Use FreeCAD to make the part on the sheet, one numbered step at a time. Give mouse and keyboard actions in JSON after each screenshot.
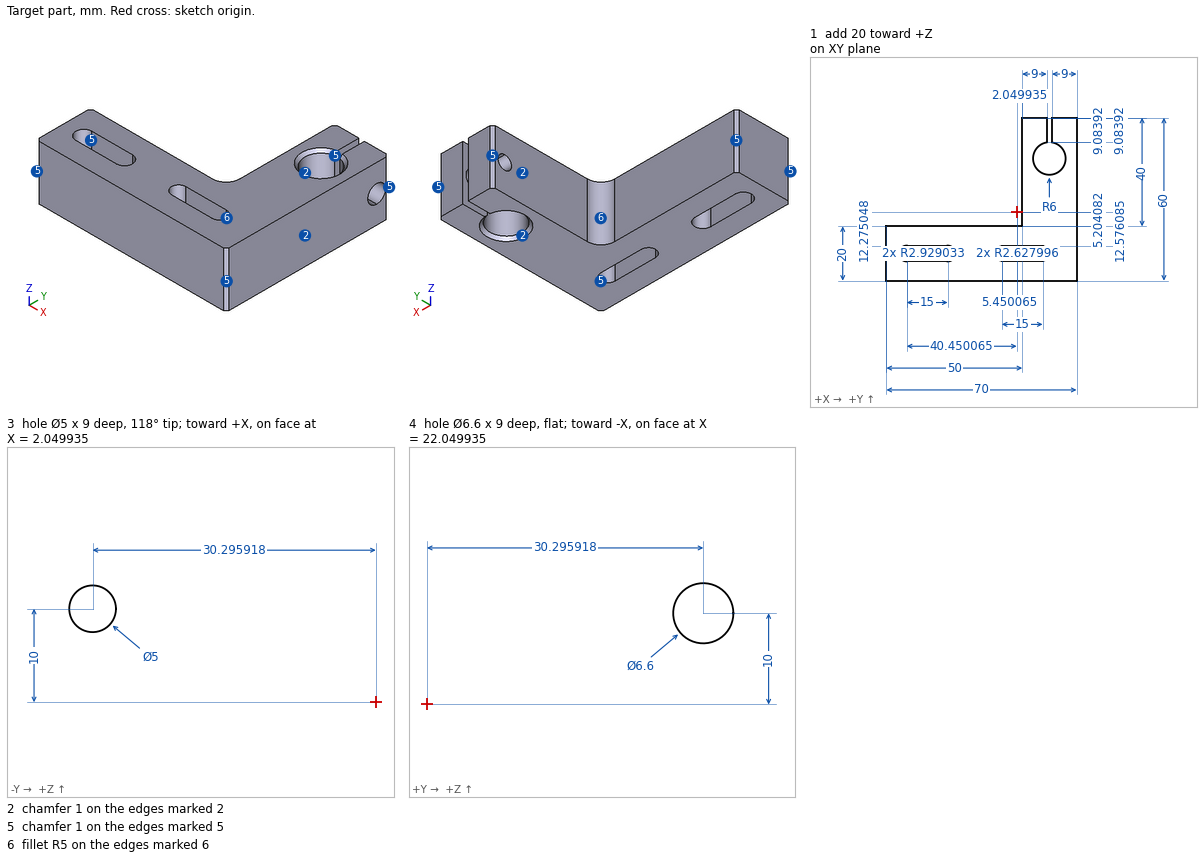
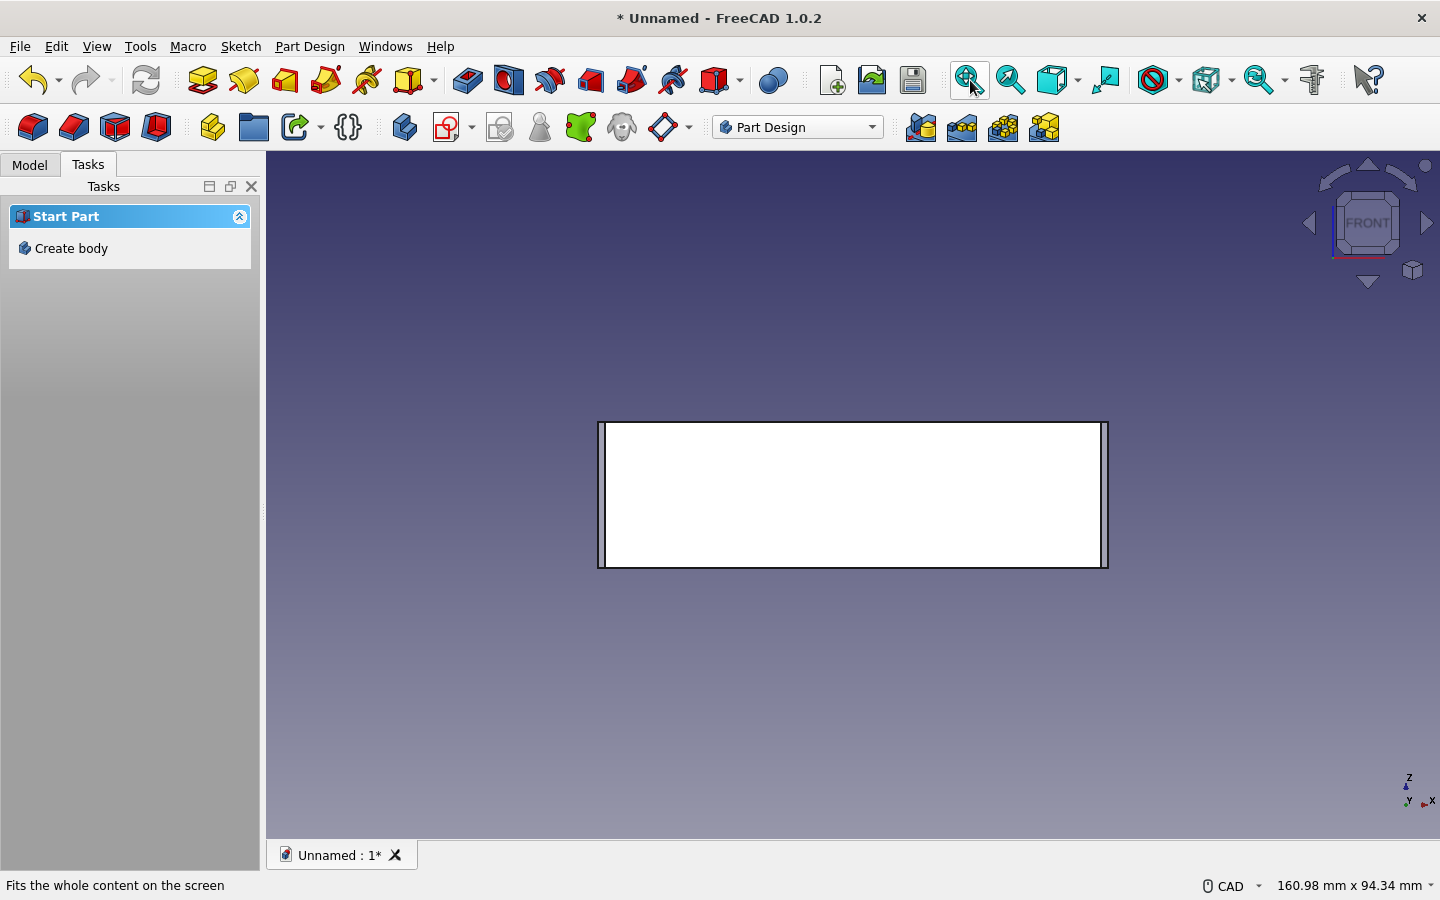
{"action": "left_click", "coordinate": [970, 80]}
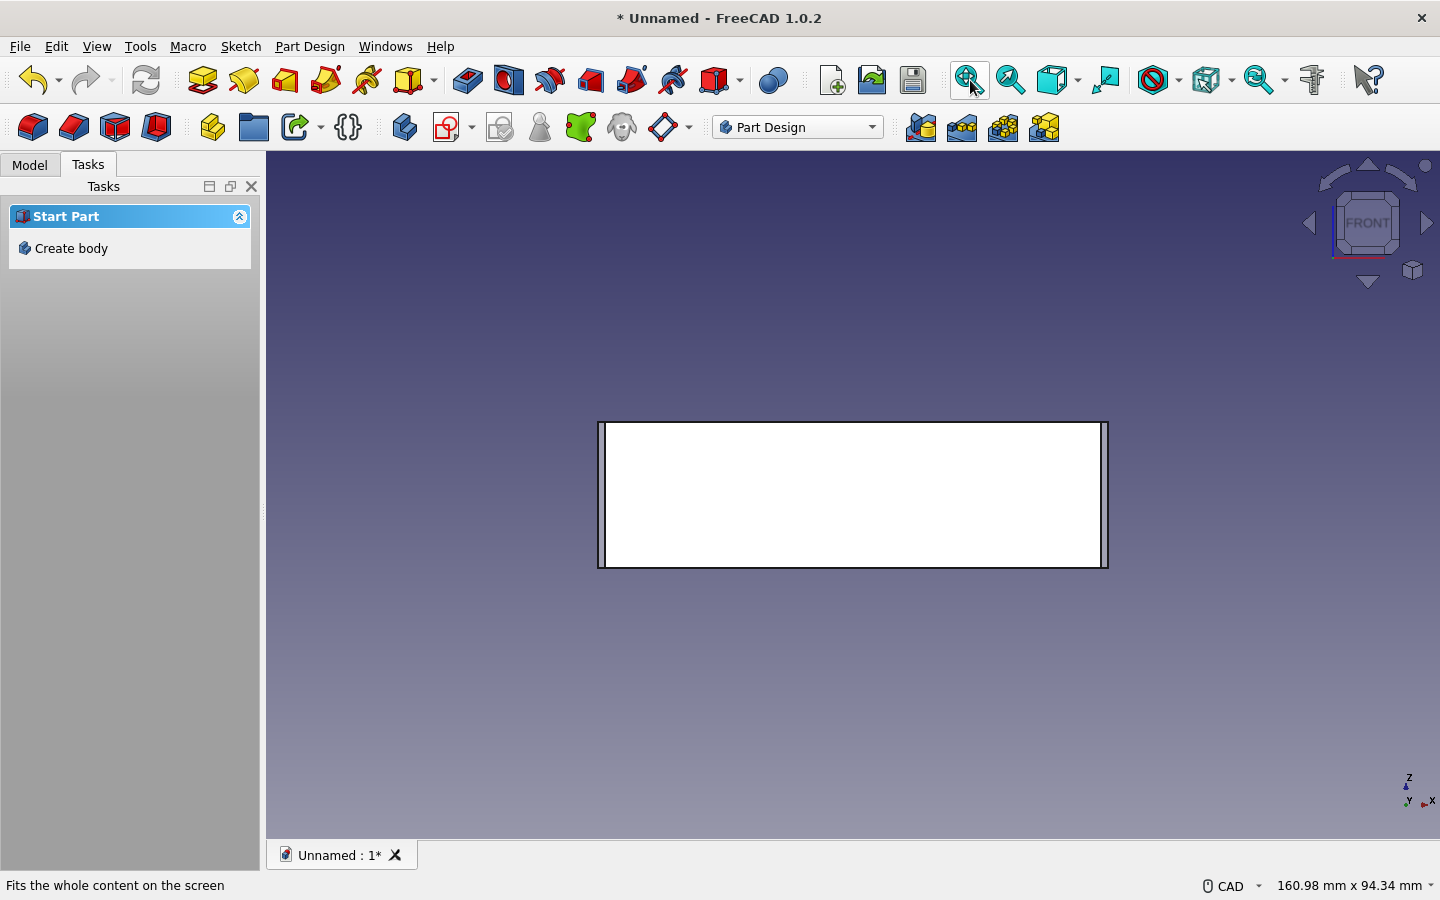
{"action": "key", "text": "3"}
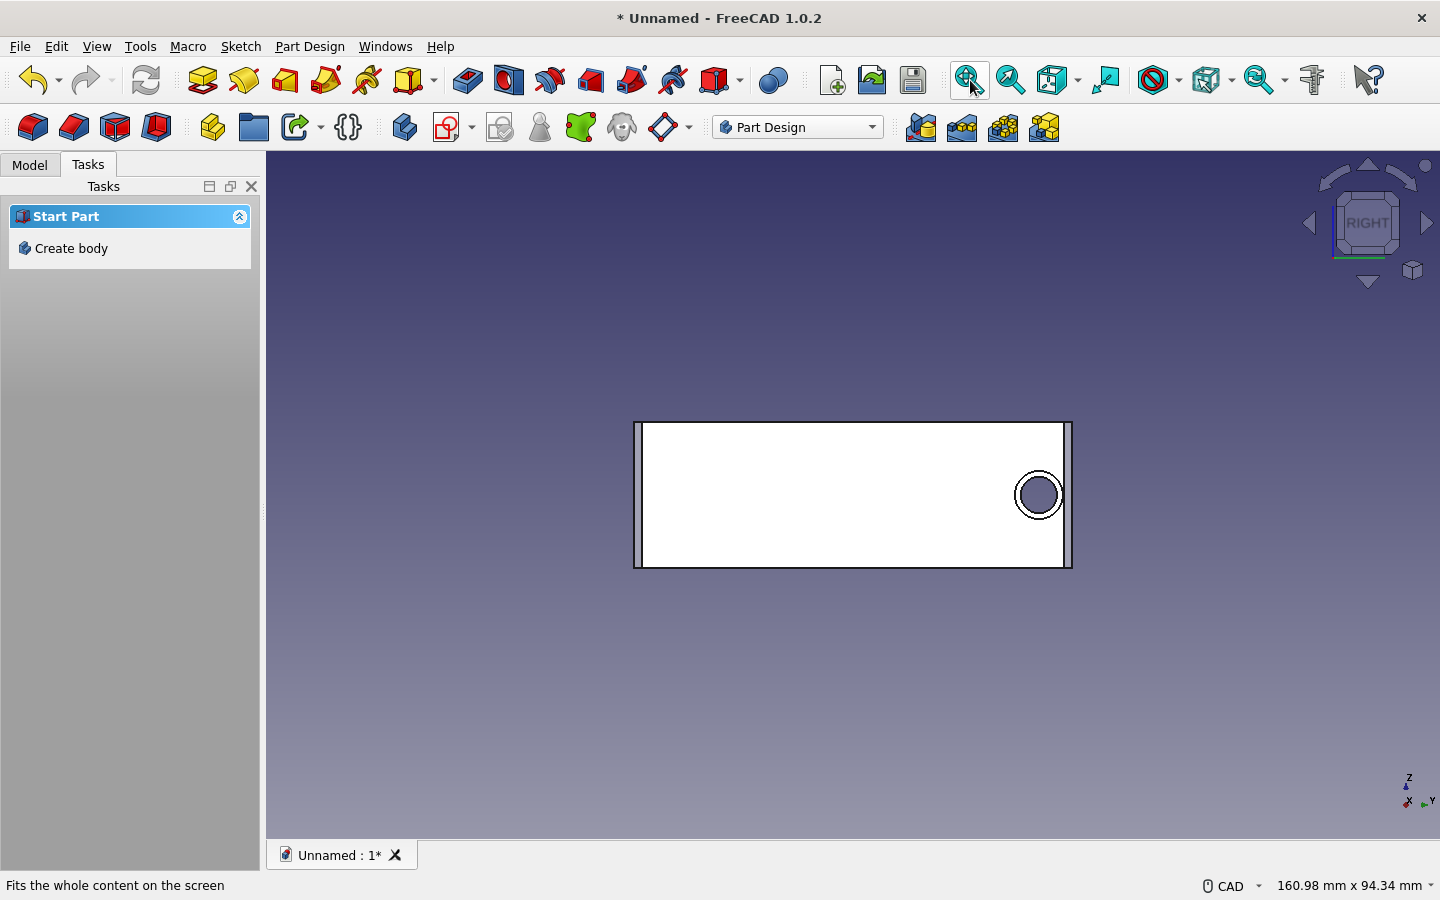
{"action": "left_click", "coordinate": [970, 80]}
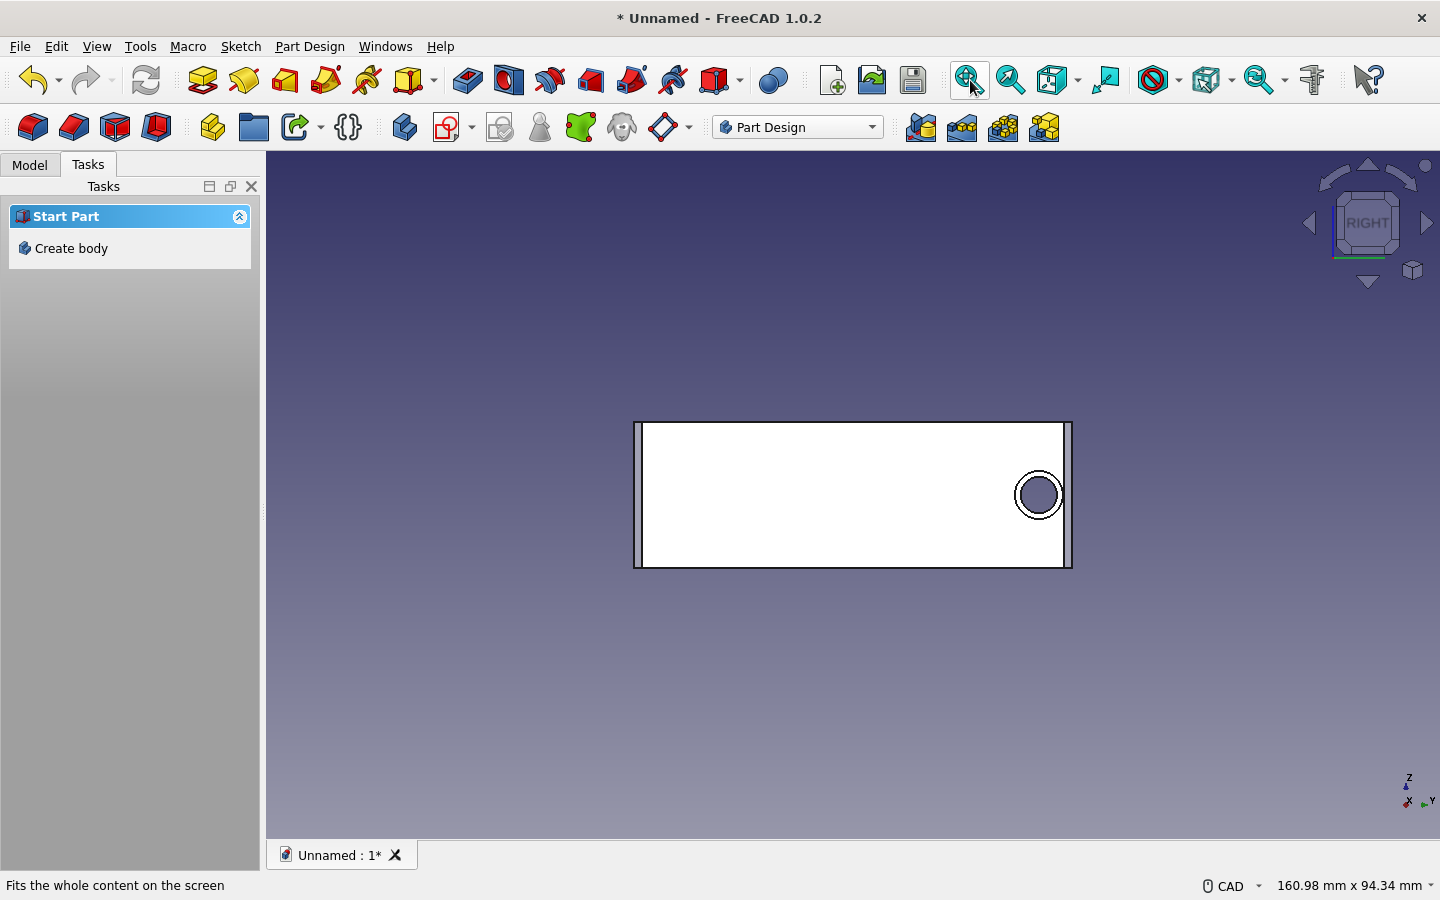
{"action": "key", "text": "5"}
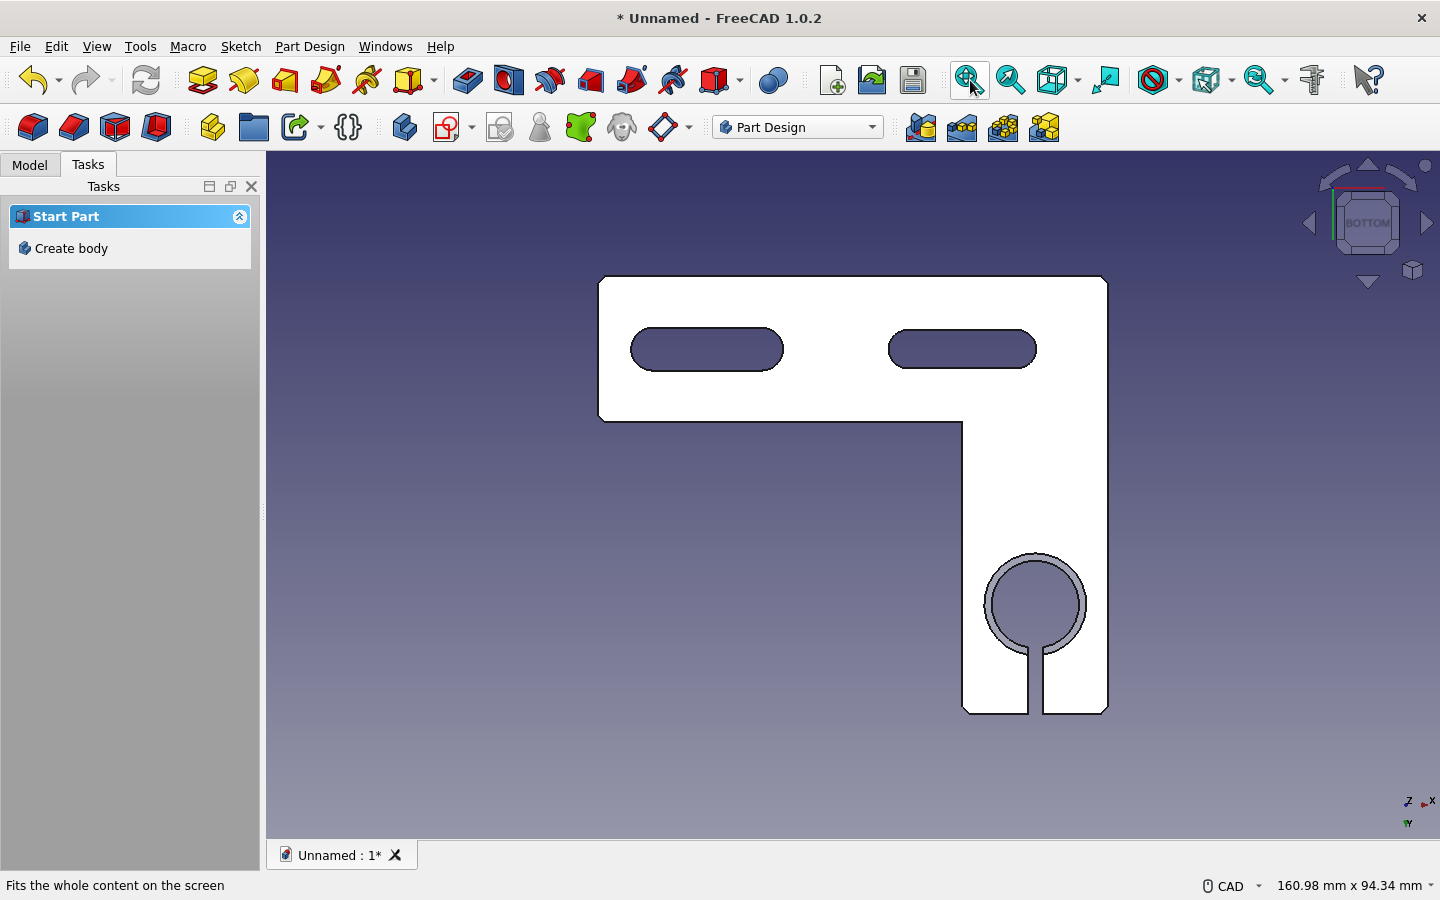
{"action": "key", "text": "4"}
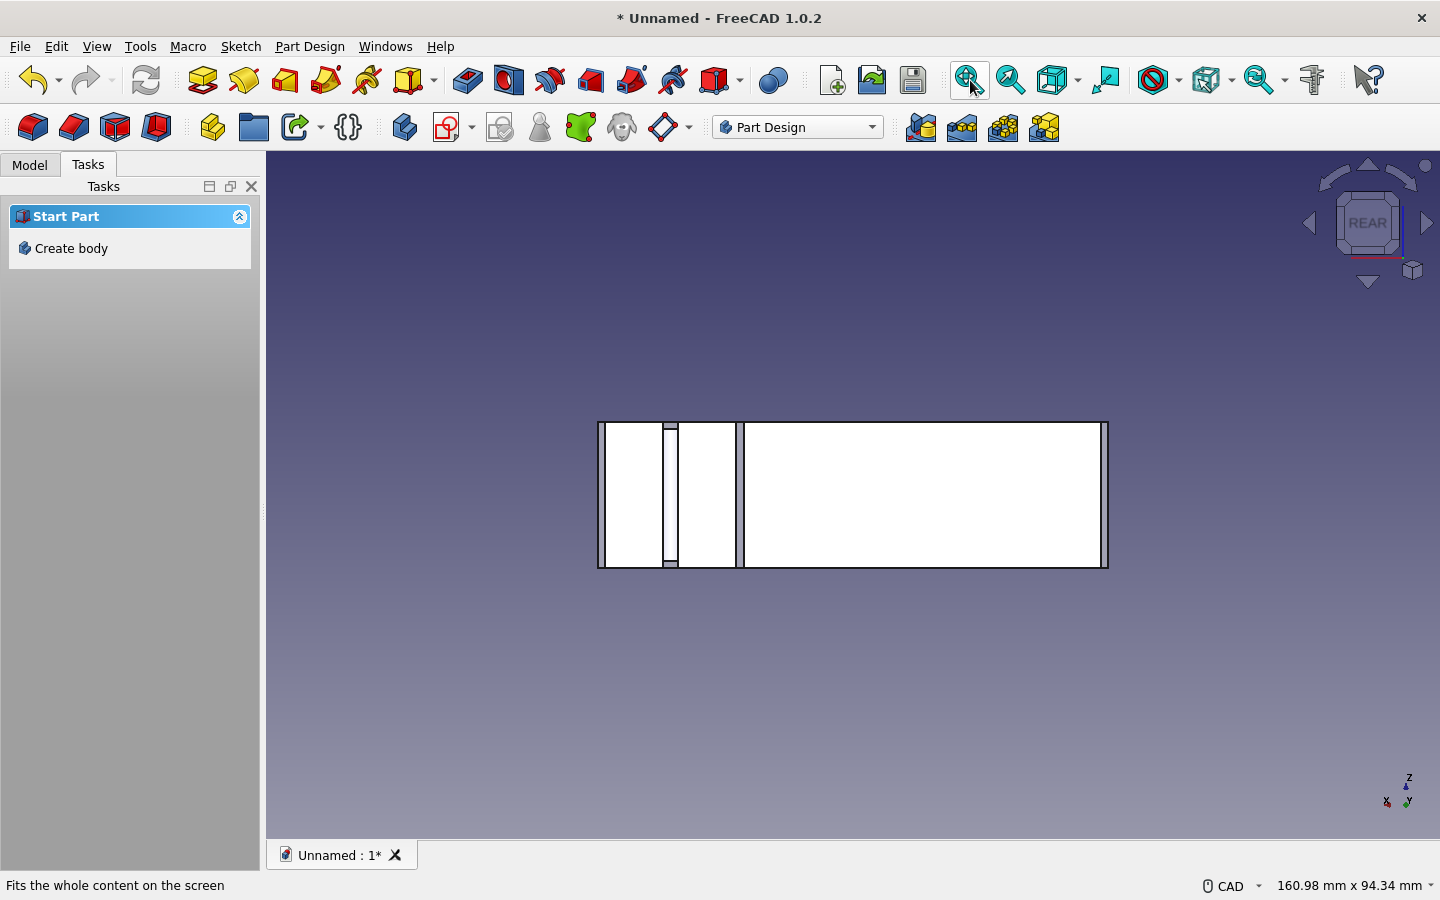
{"action": "left_click", "coordinate": [970, 80]}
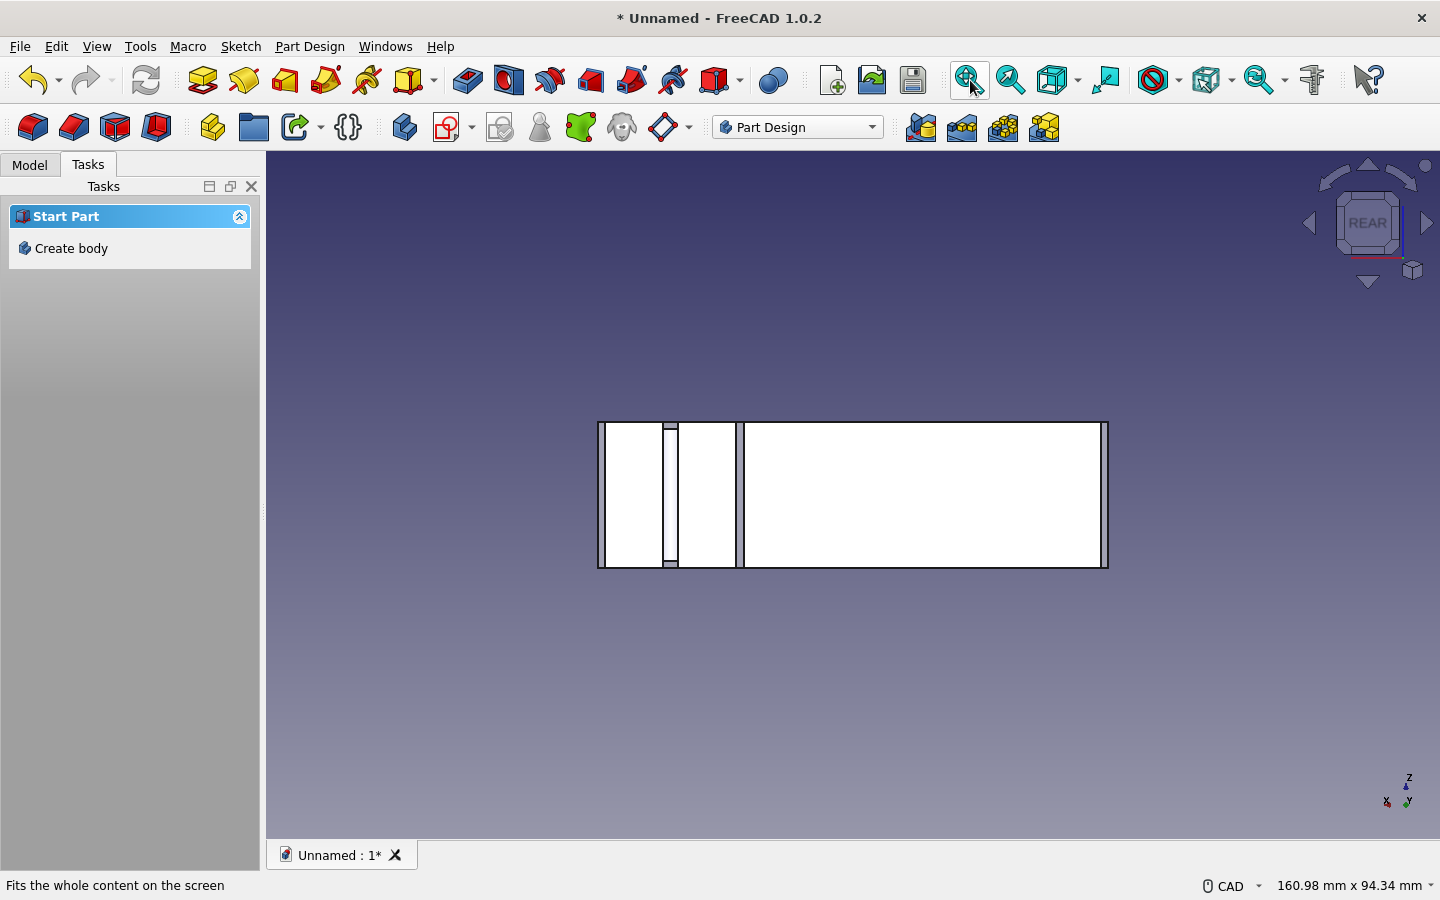
{"action": "key", "text": "6"}